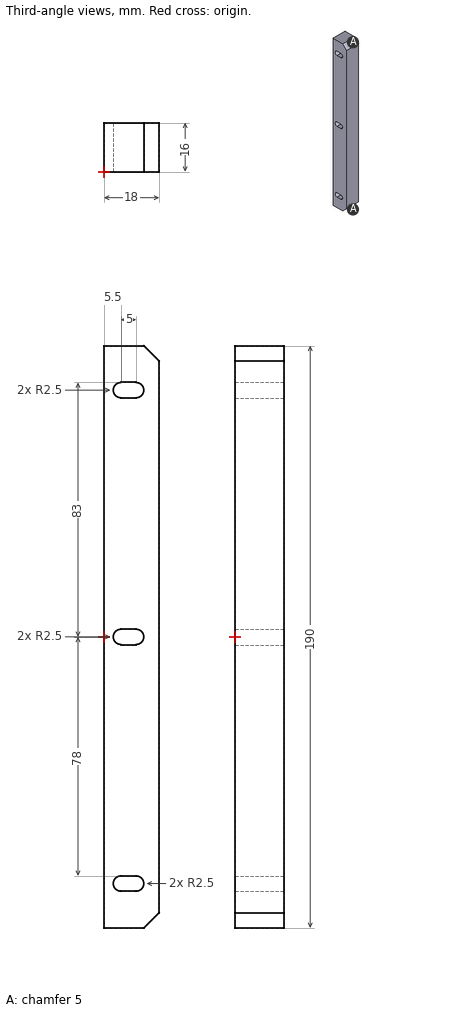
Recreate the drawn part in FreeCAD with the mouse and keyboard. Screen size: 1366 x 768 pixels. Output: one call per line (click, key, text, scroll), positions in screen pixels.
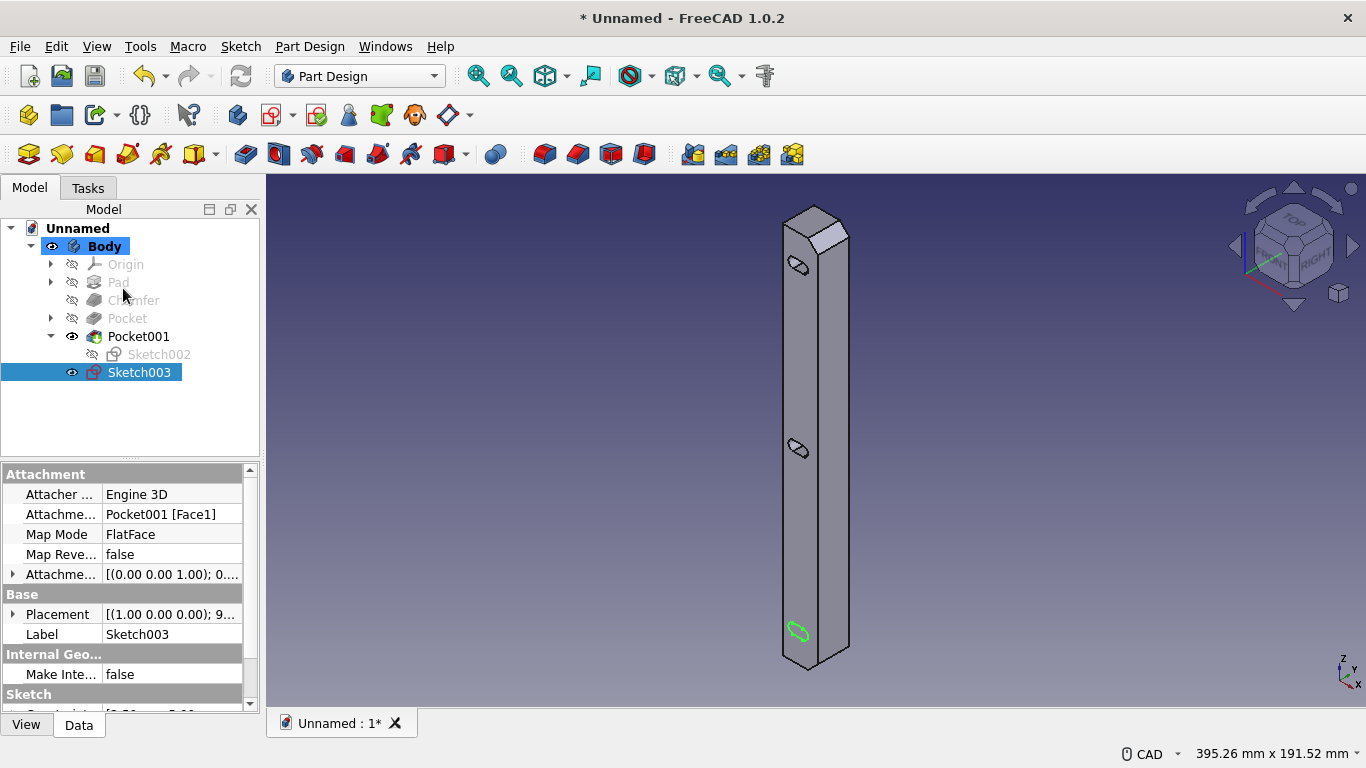
click(246, 154)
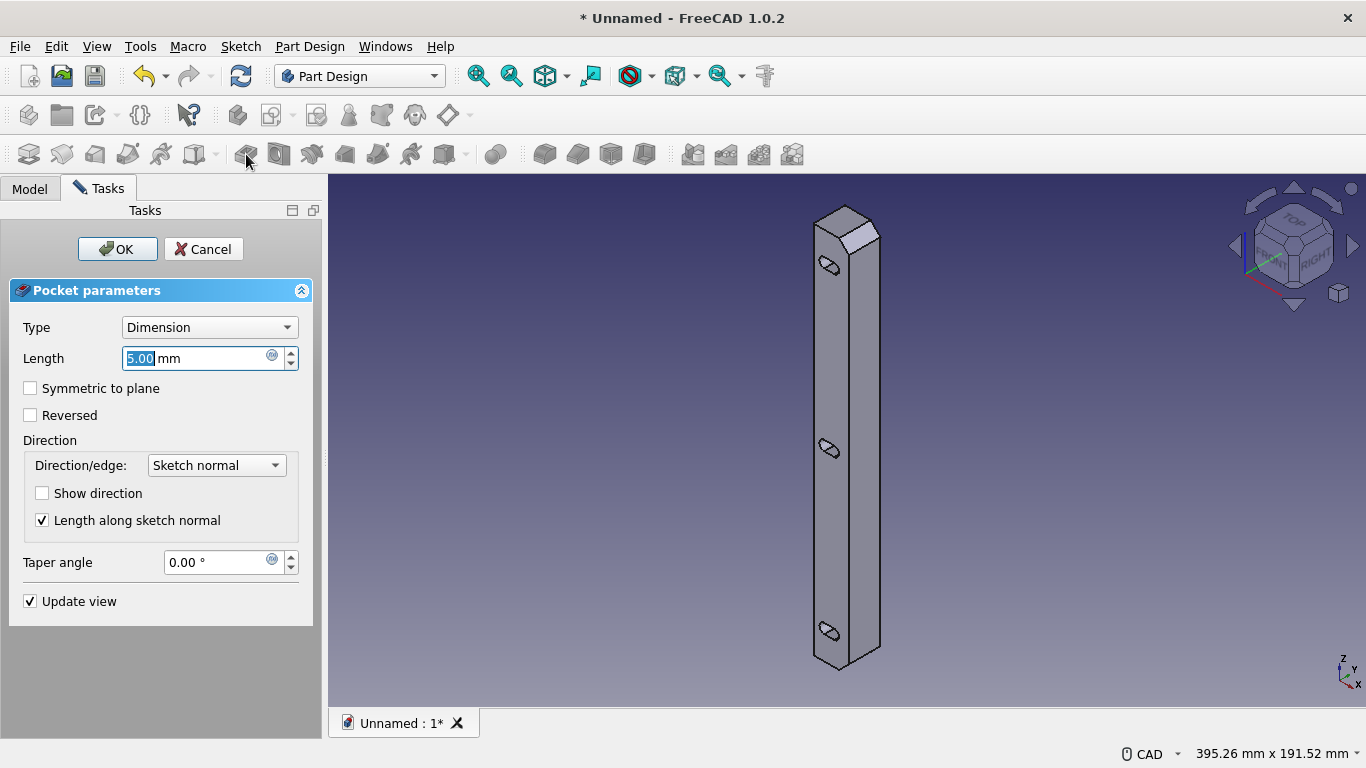
click(210, 328)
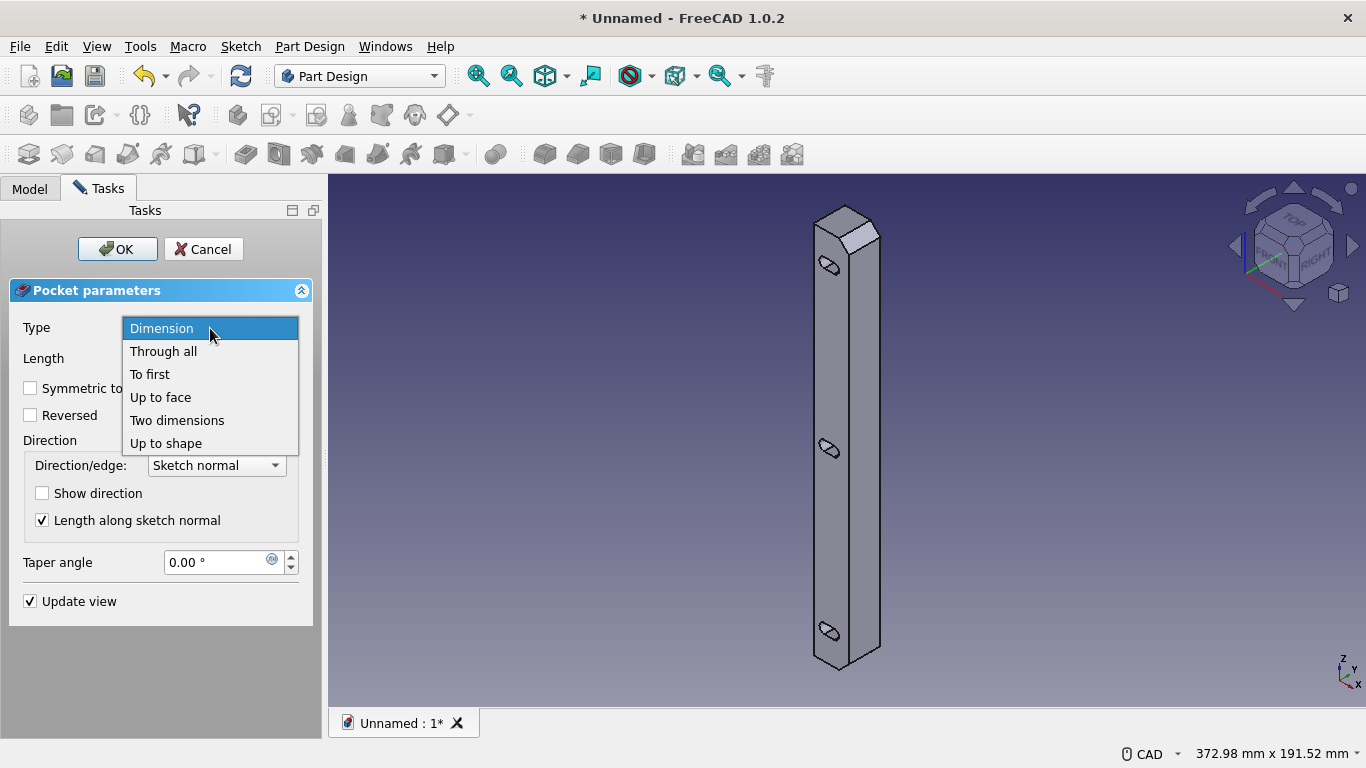
click(208, 374)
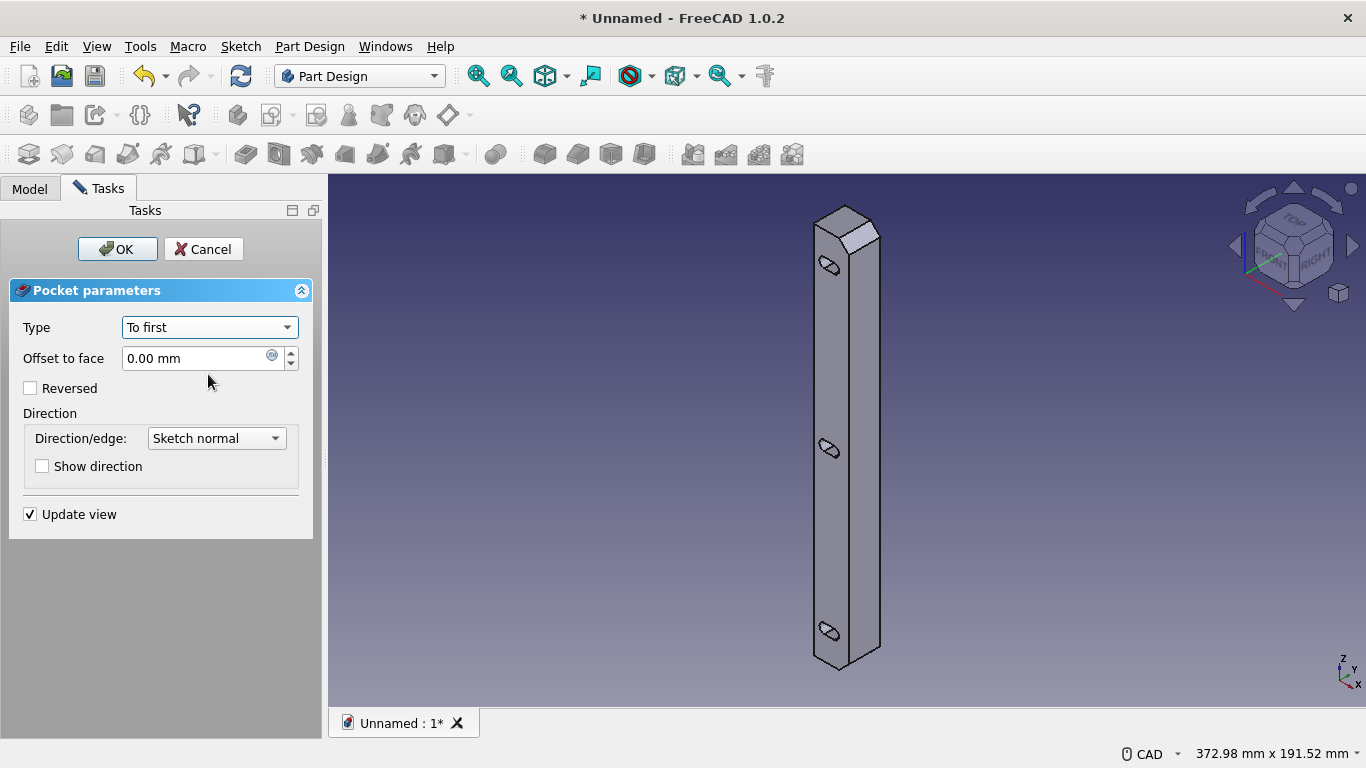
click(118, 249)